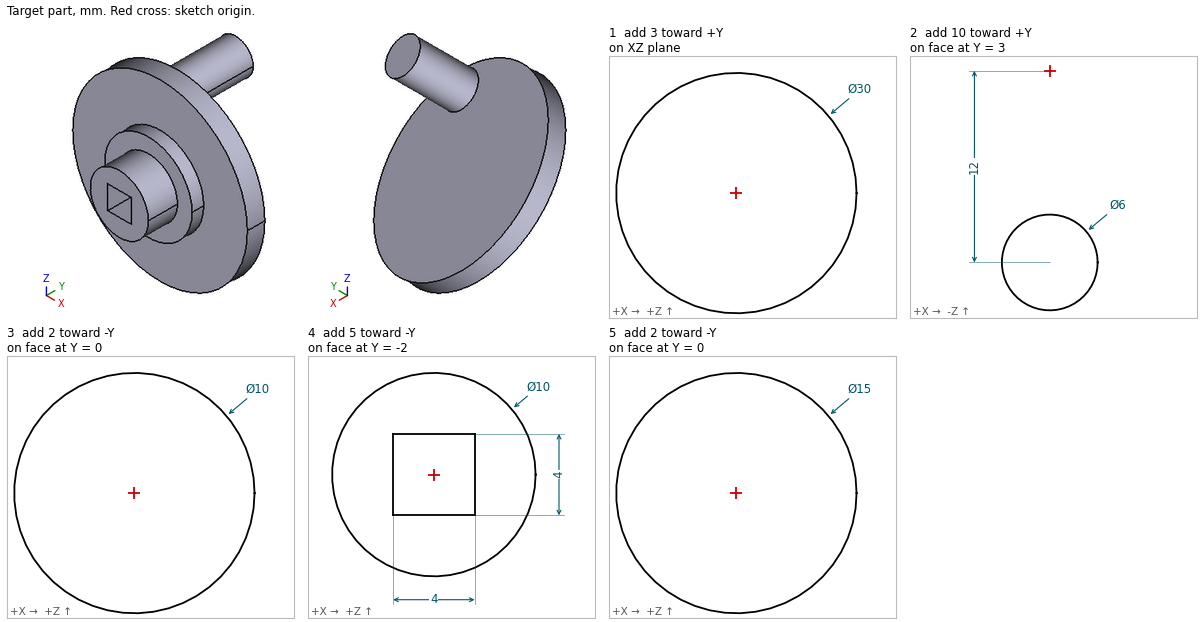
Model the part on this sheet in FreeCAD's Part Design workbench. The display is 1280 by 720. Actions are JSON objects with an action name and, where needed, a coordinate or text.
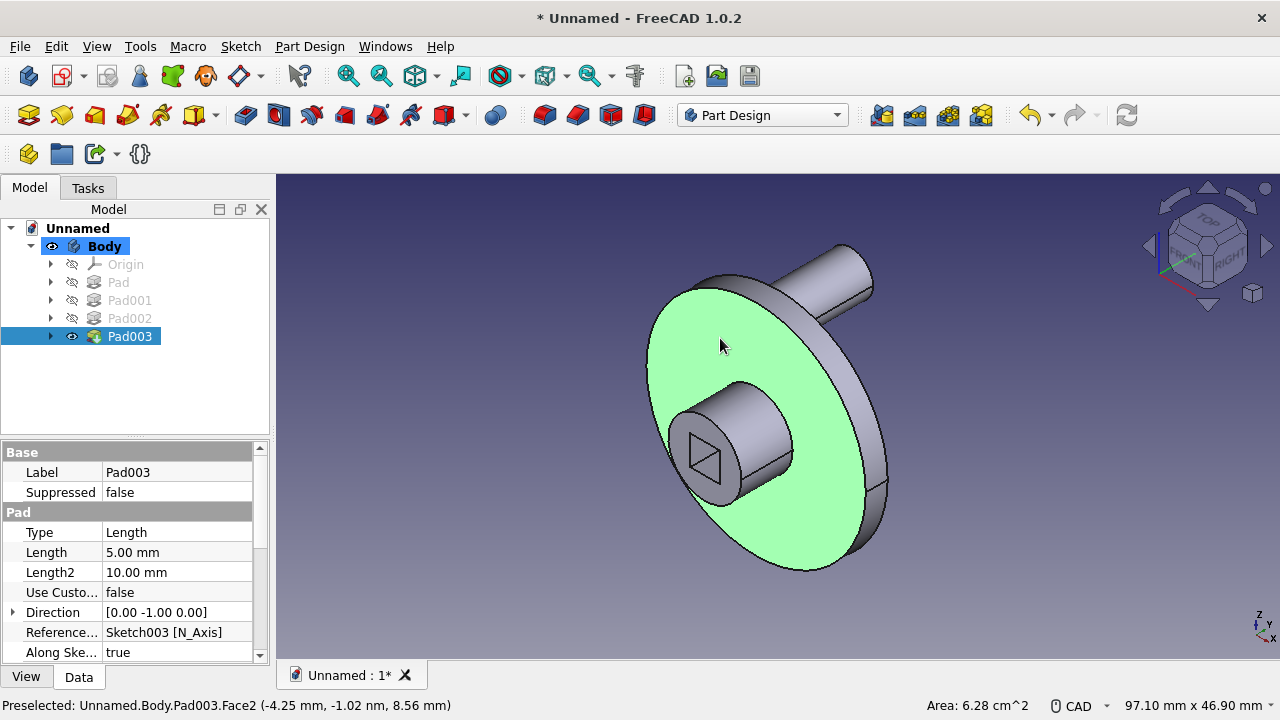
{"action": "left_click", "coordinate": [62, 76]}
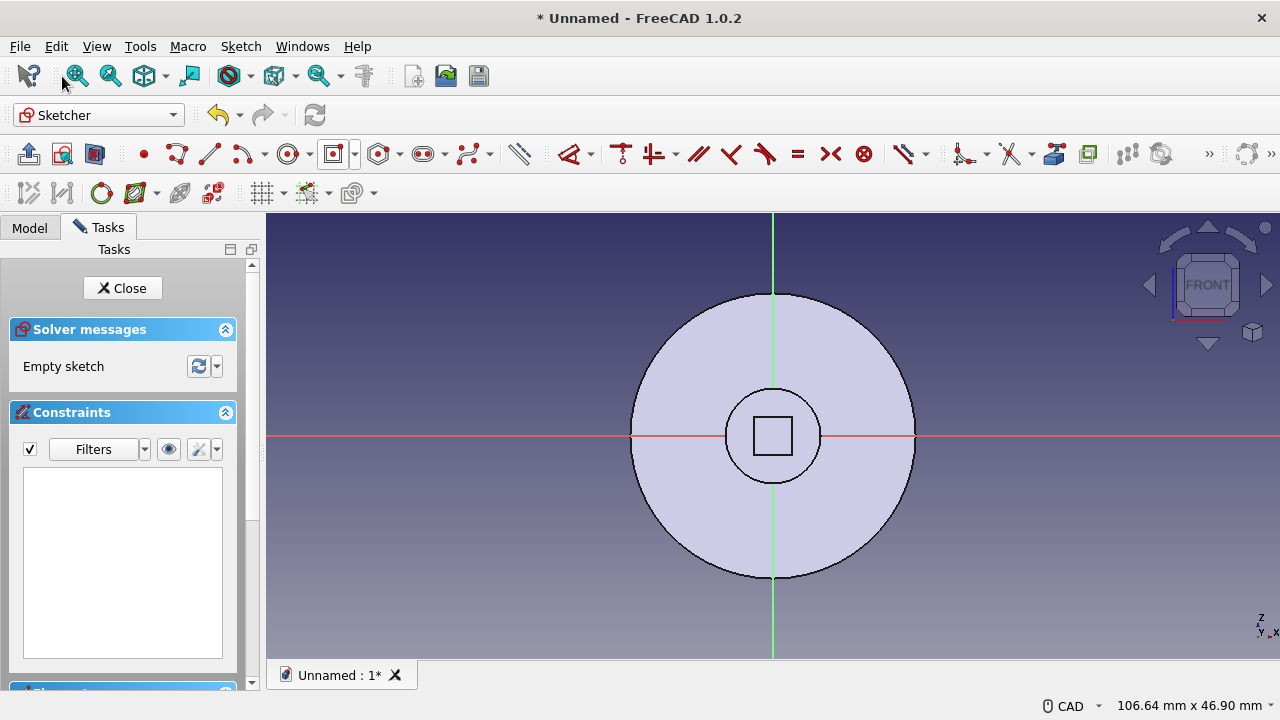
{"action": "scroll", "coordinate": [856, 436], "scroll_direction": "up", "scroll_amount": 3}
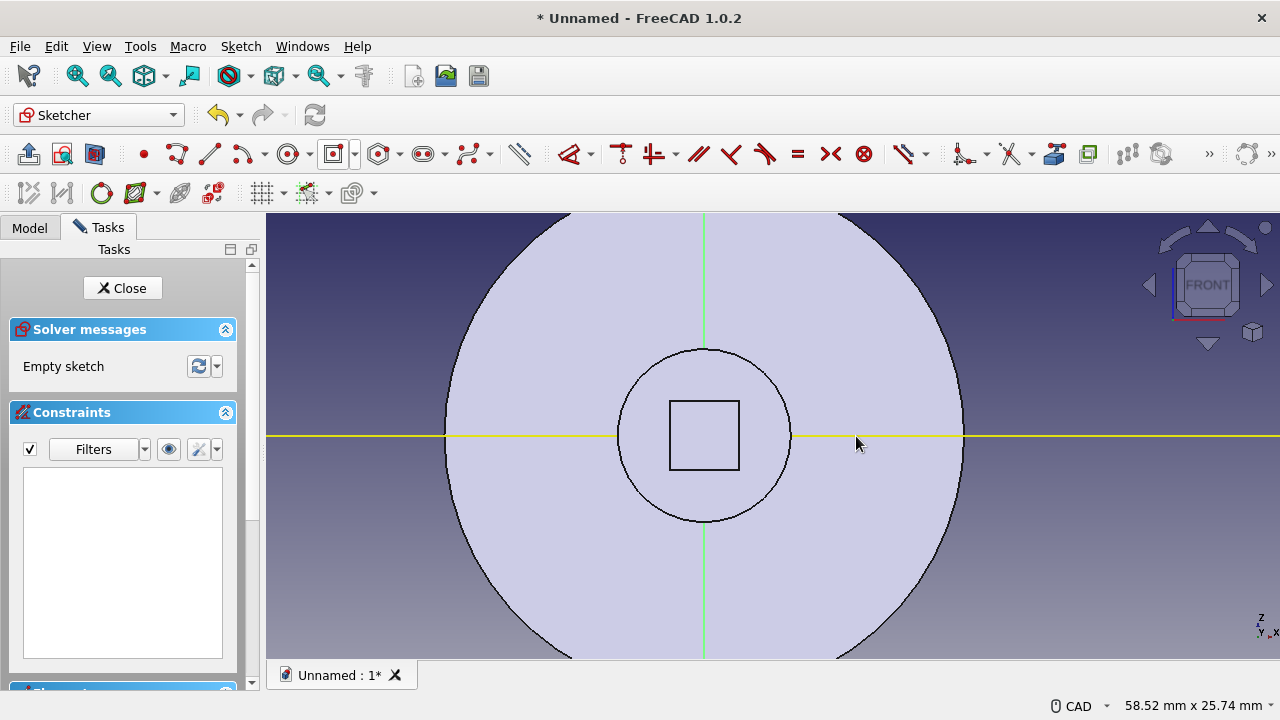
{"action": "left_click", "coordinate": [288, 154]}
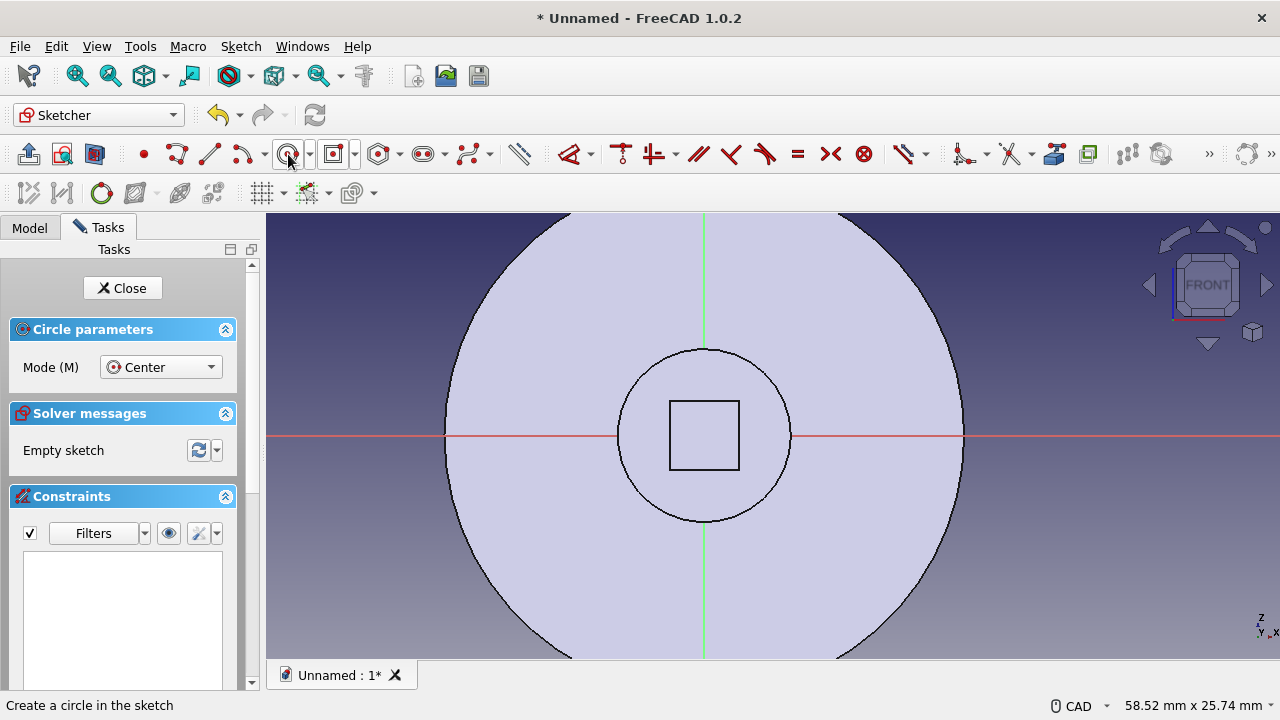
{"action": "left_click", "coordinate": [704, 436]}
{"action": "left_click", "coordinate": [796, 344]}
{"action": "key", "text": "Escape"}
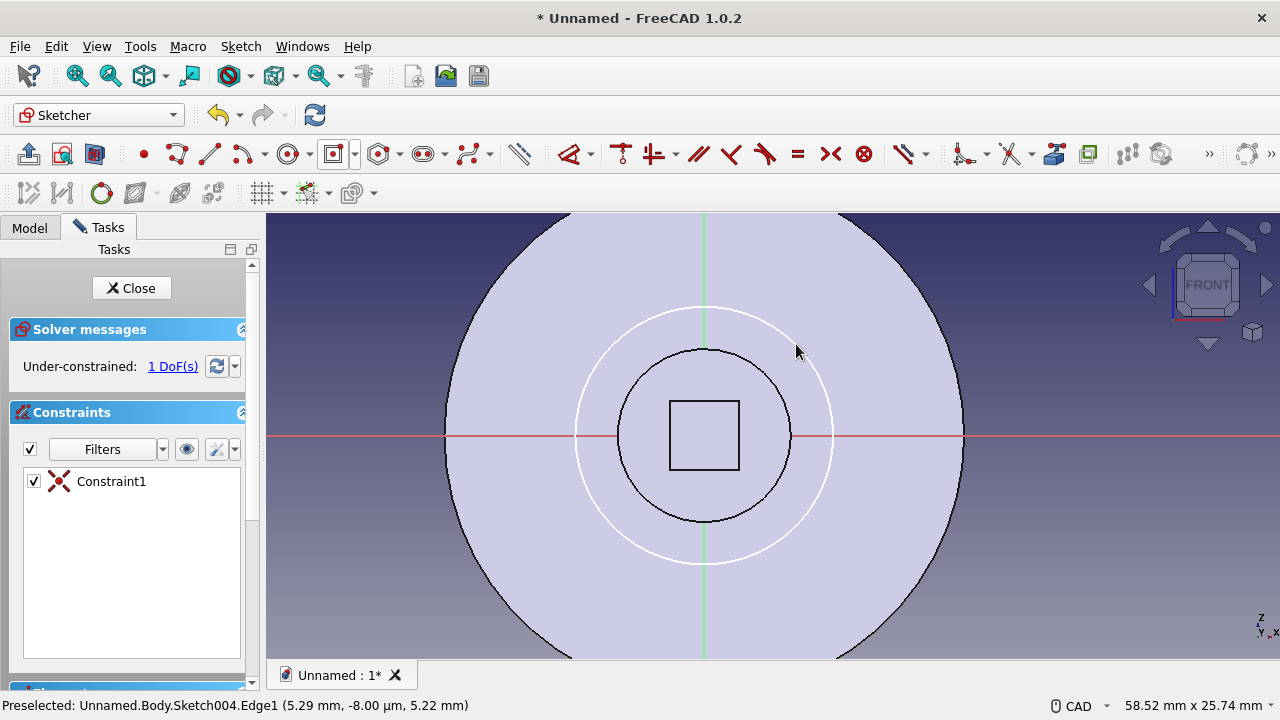
{"action": "left_click", "coordinate": [568, 154]}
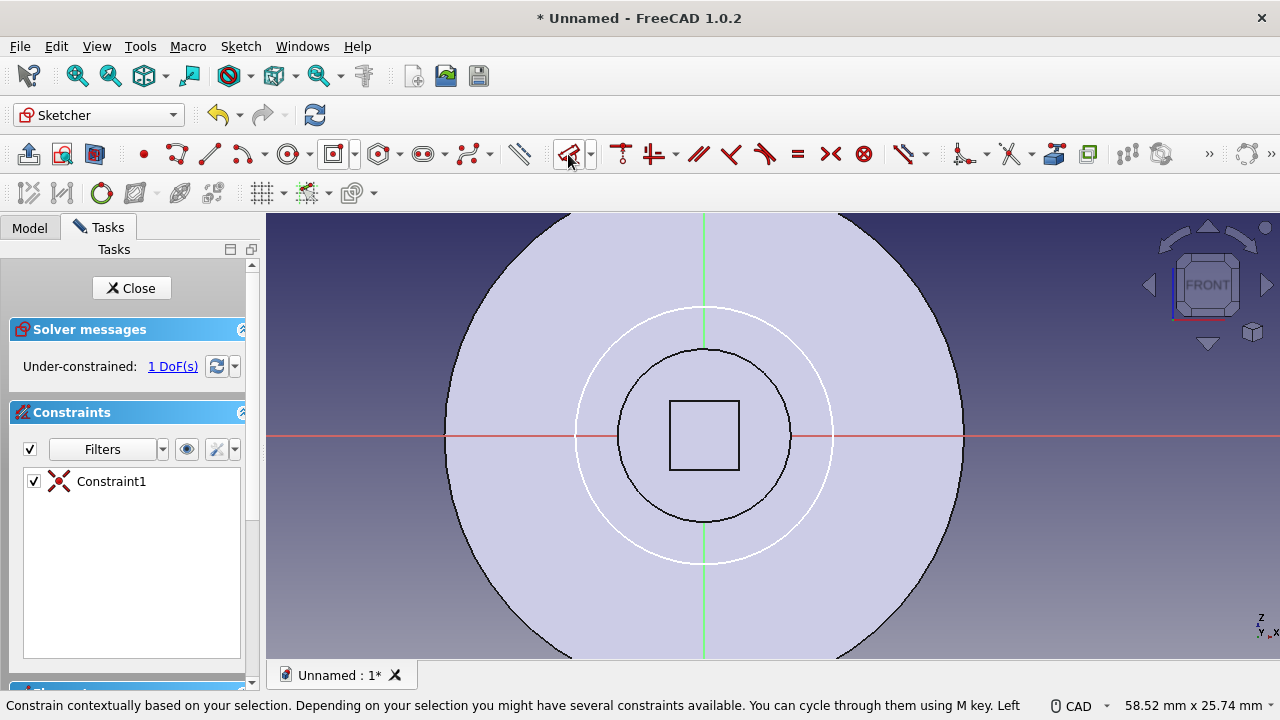
{"action": "left_click", "coordinate": [795, 344]}
{"action": "left_click", "coordinate": [818, 321]}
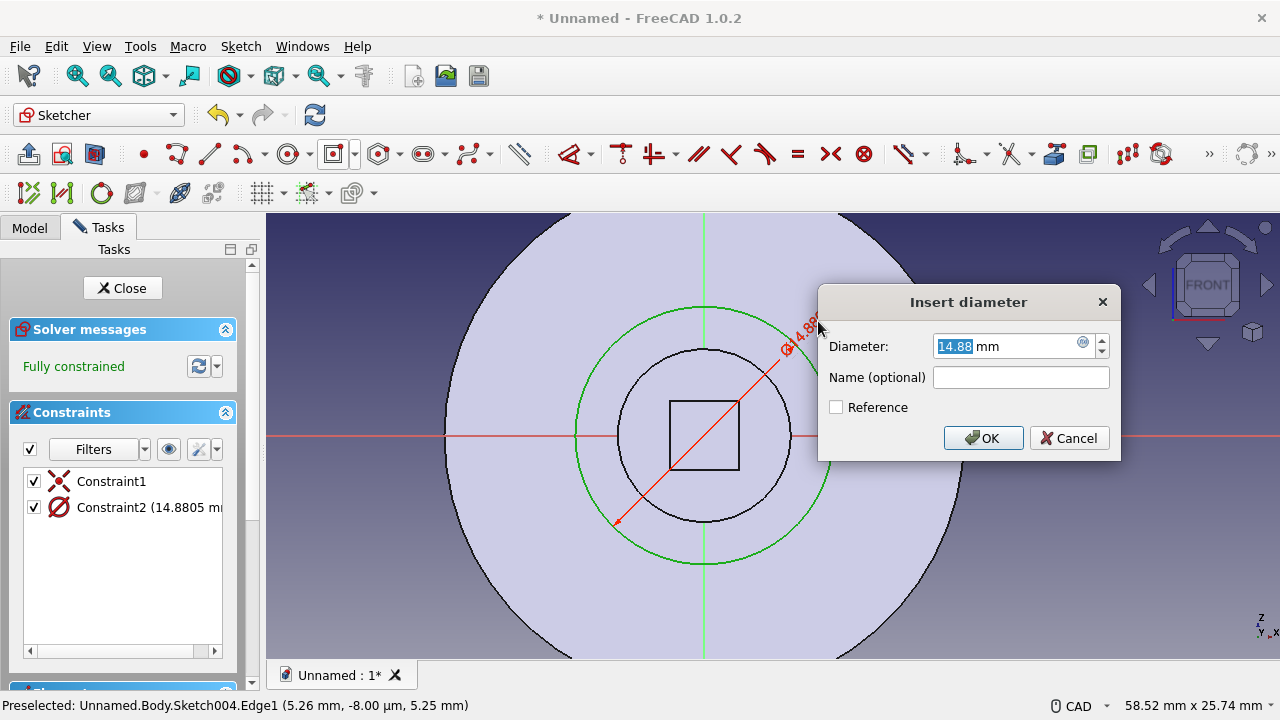
{"action": "type", "text": "15"}
{"action": "key", "text": "Return"}
{"action": "key", "text": "Escape"}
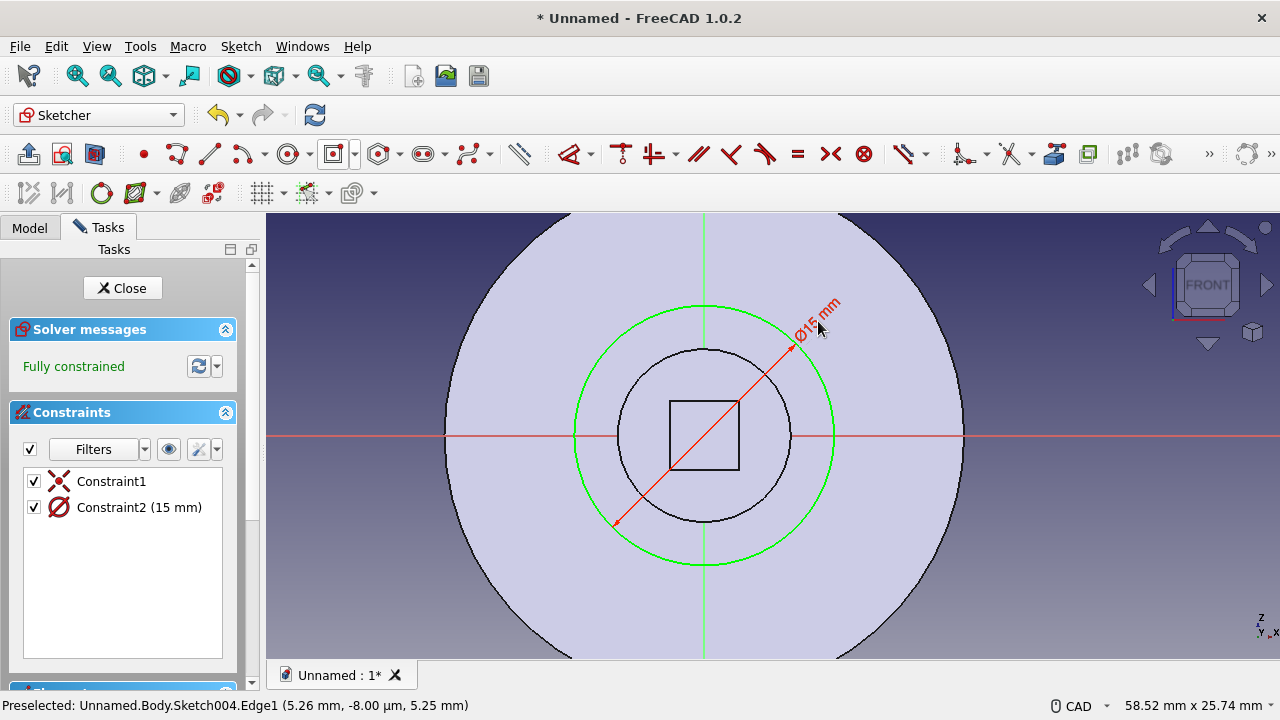
{"action": "left_click", "coordinate": [123, 288]}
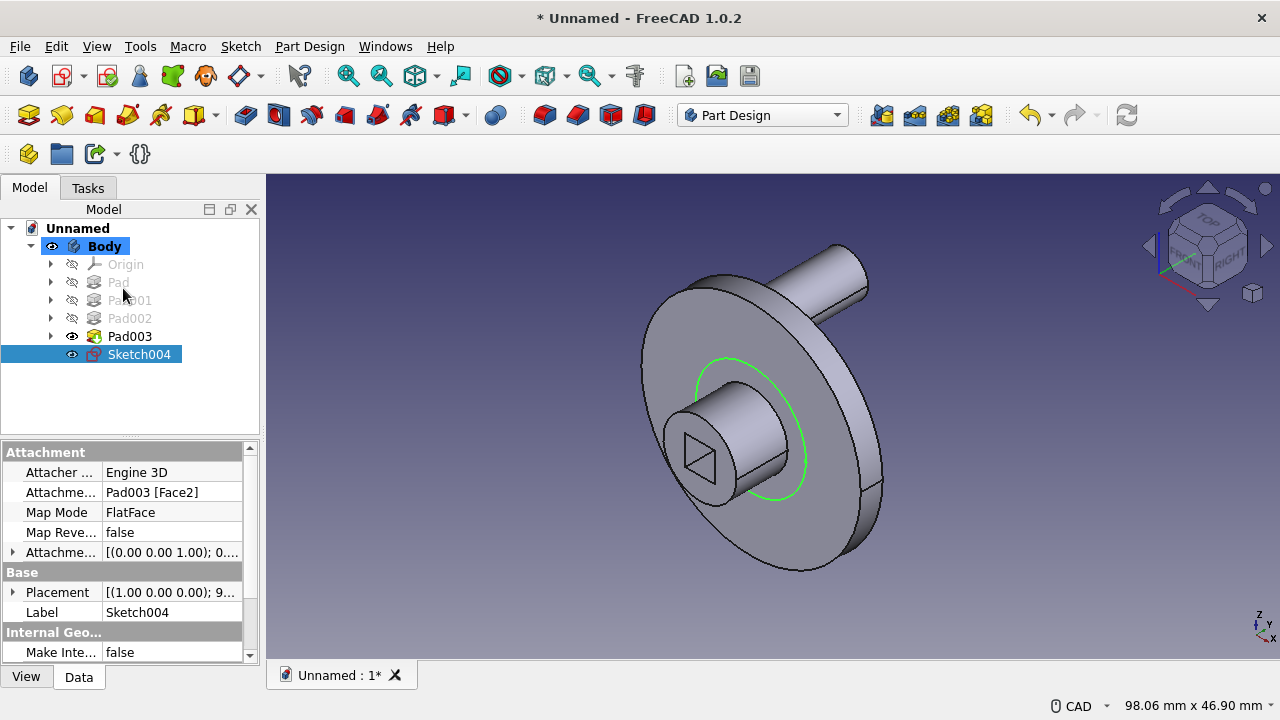
{"action": "left_click", "coordinate": [29, 116]}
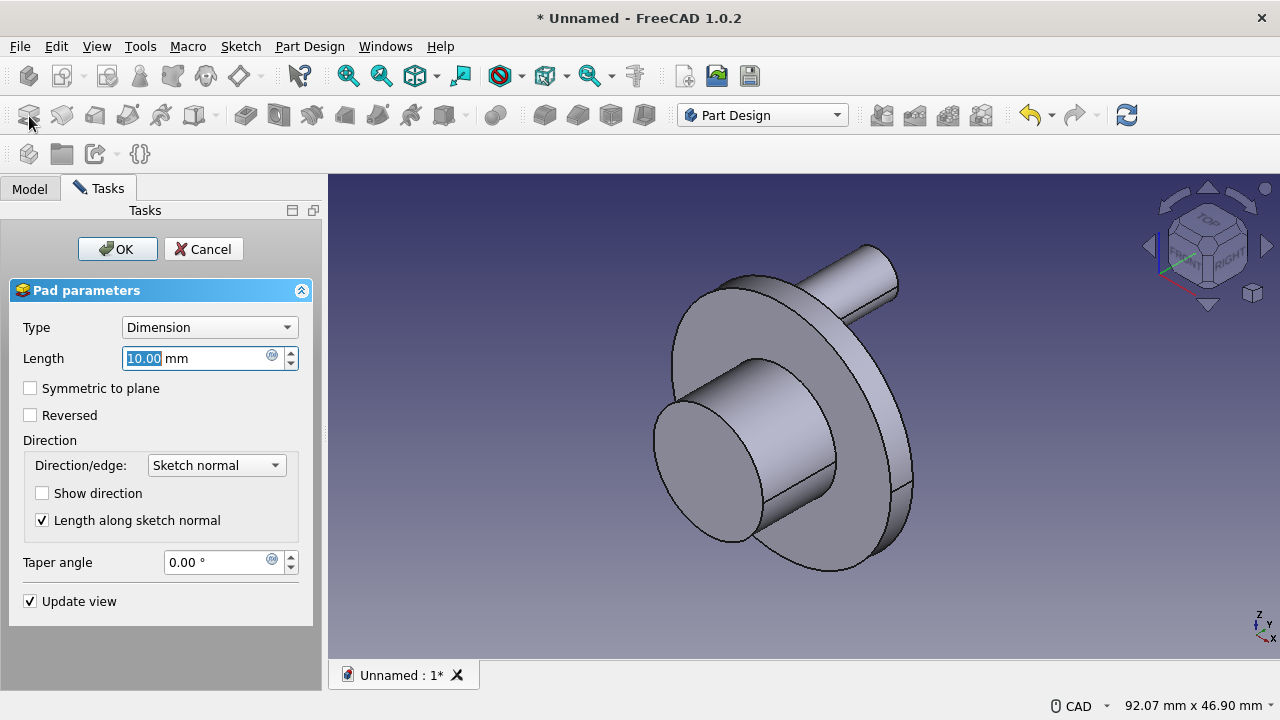
{"action": "type", "text": "2"}
{"action": "key", "text": "Tab"}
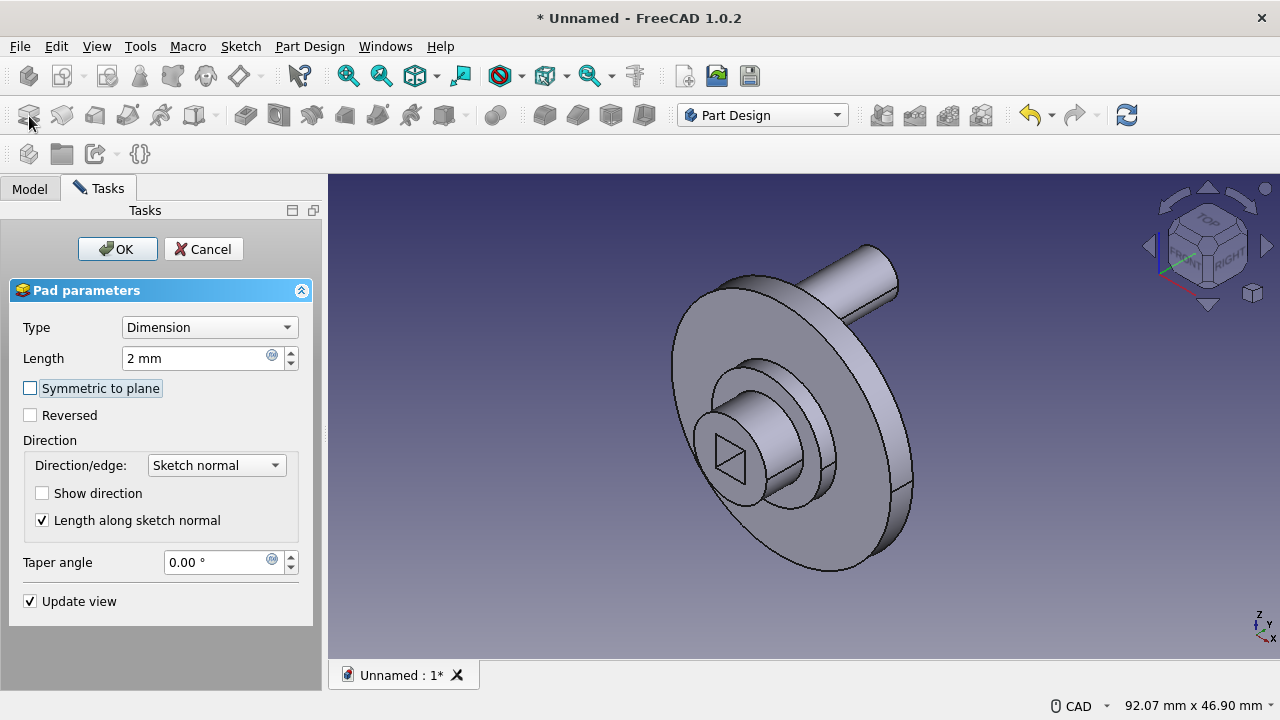
{"action": "left_click", "coordinate": [118, 249]}